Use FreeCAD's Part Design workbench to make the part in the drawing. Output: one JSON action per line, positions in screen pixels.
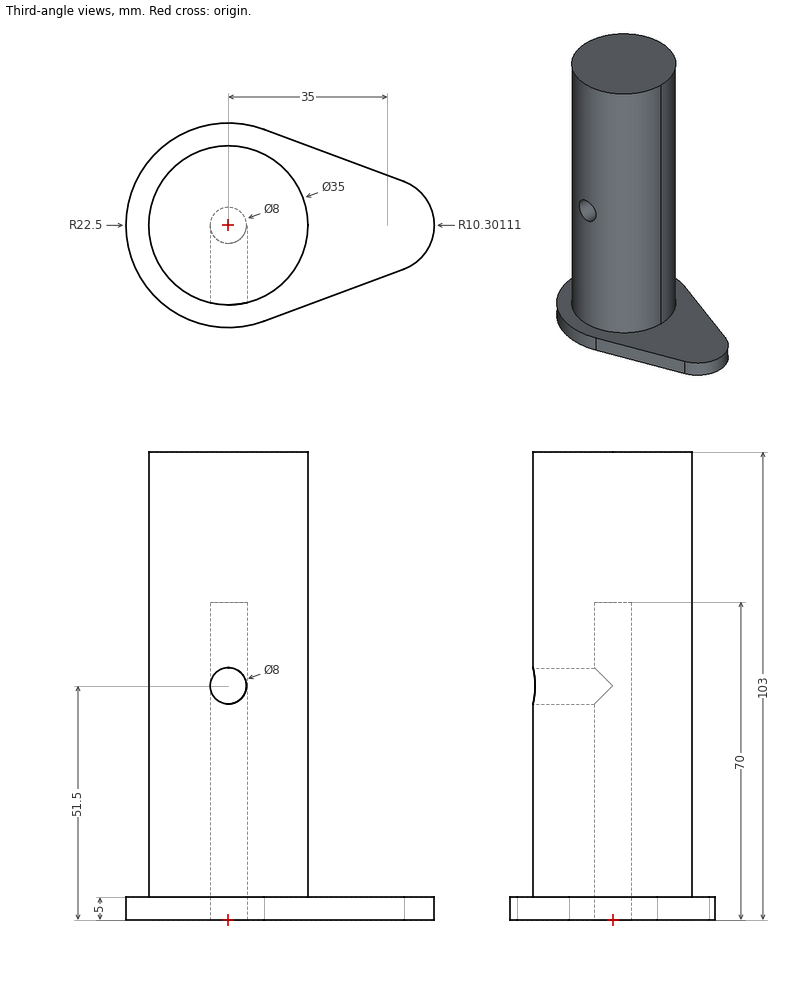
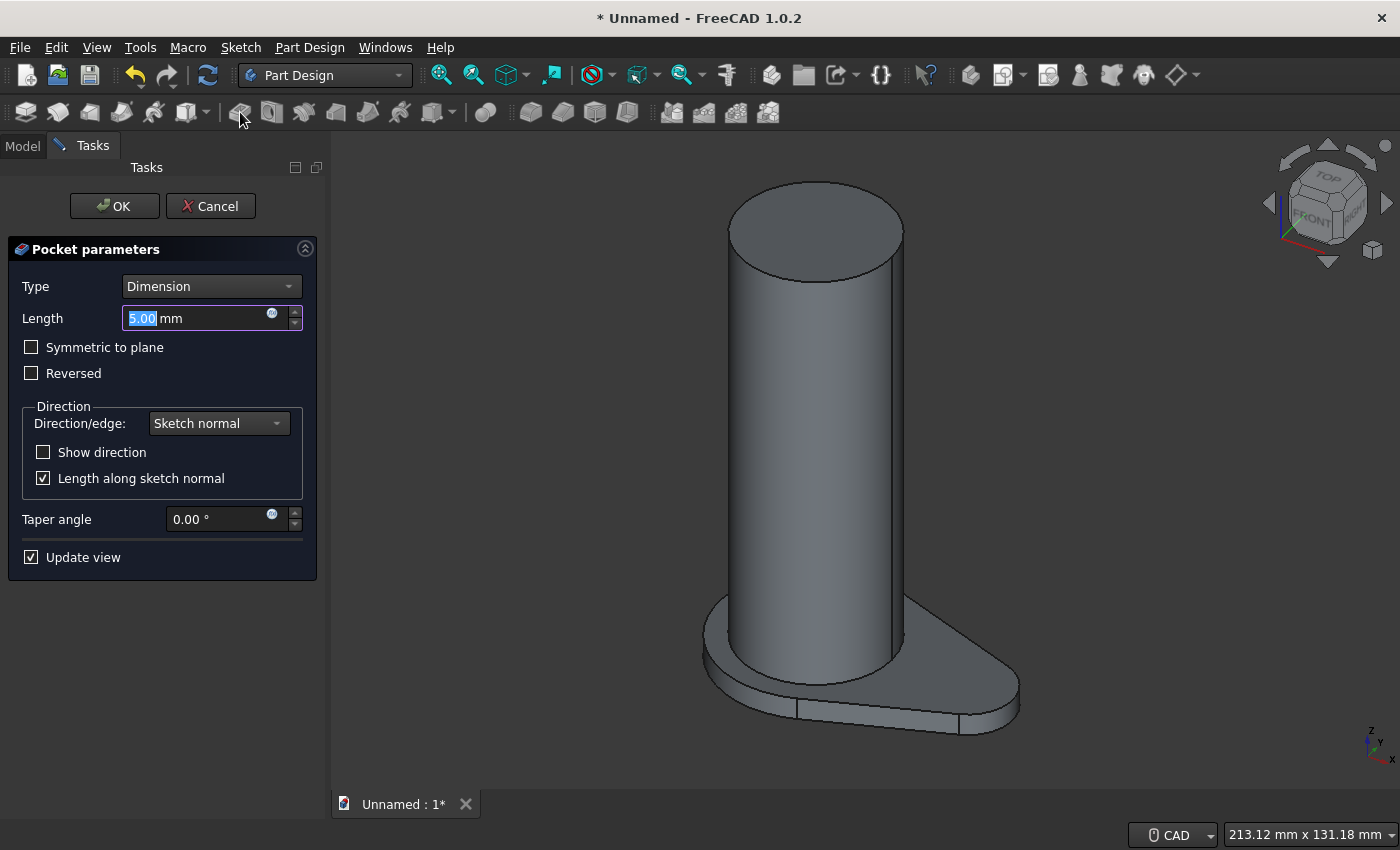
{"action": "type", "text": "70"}
{"action": "key", "text": "Tab"}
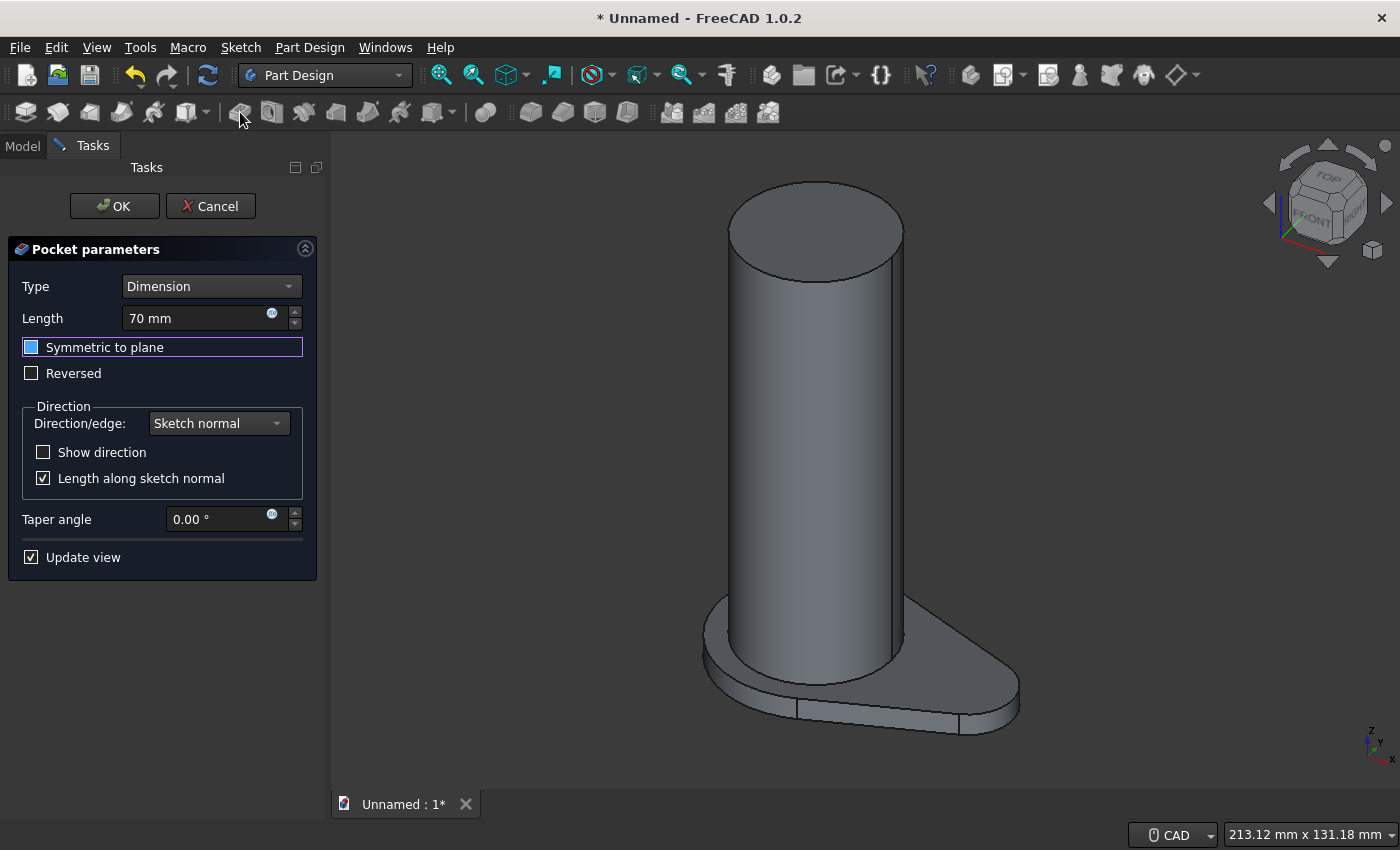
{"action": "left_click", "coordinate": [30, 373]}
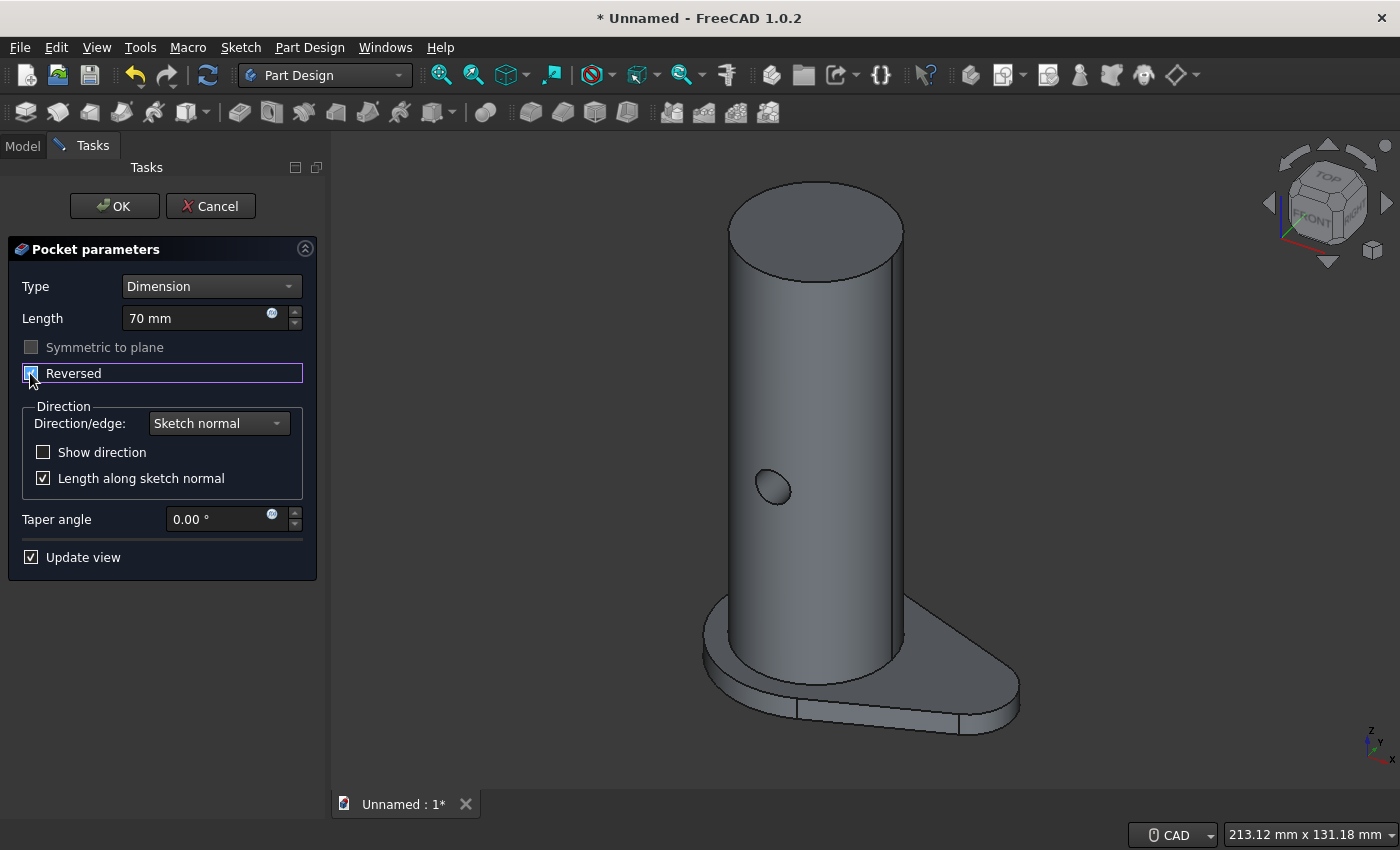
{"action": "left_click", "coordinate": [115, 206]}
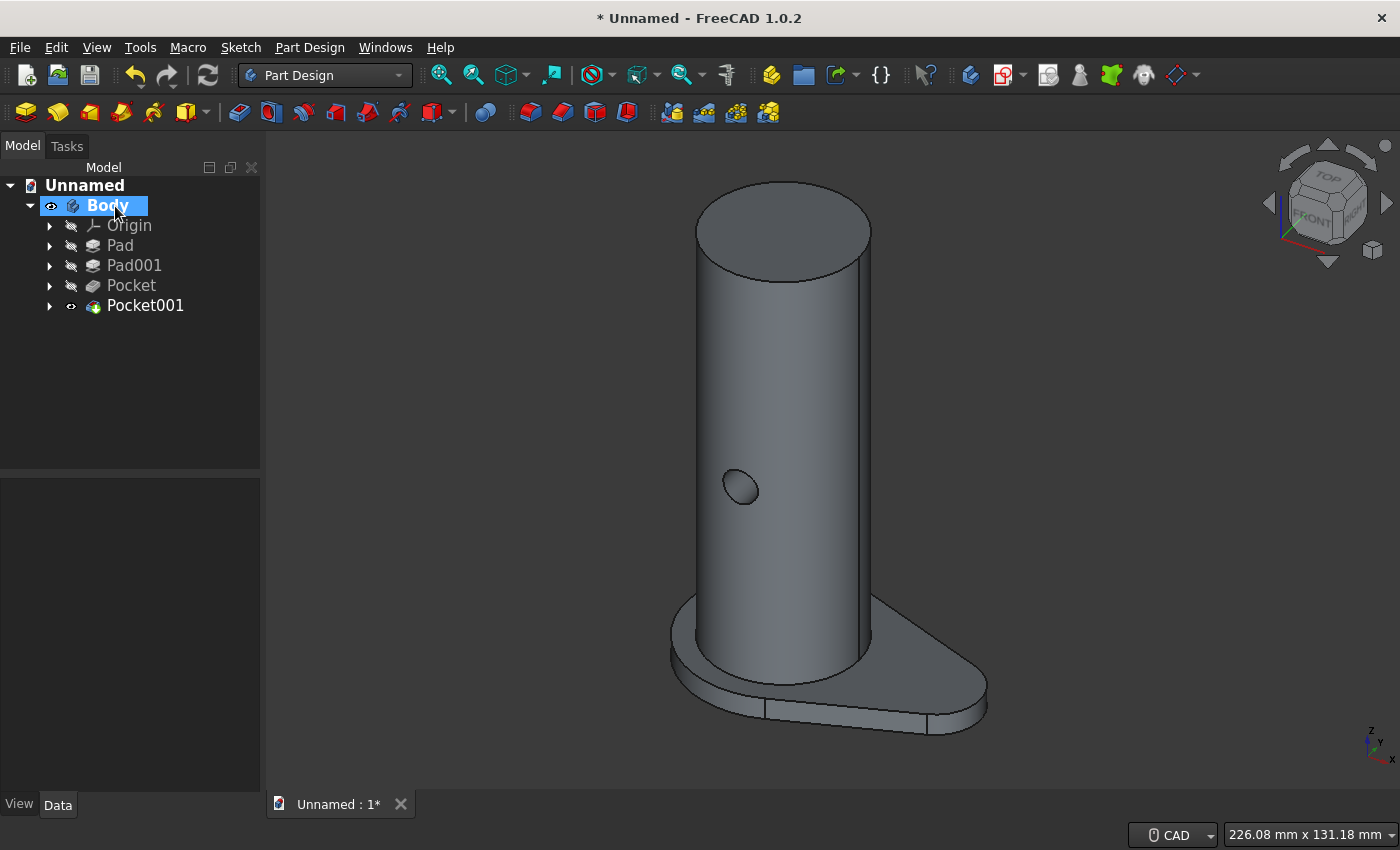
{"action": "key", "text": "0"}